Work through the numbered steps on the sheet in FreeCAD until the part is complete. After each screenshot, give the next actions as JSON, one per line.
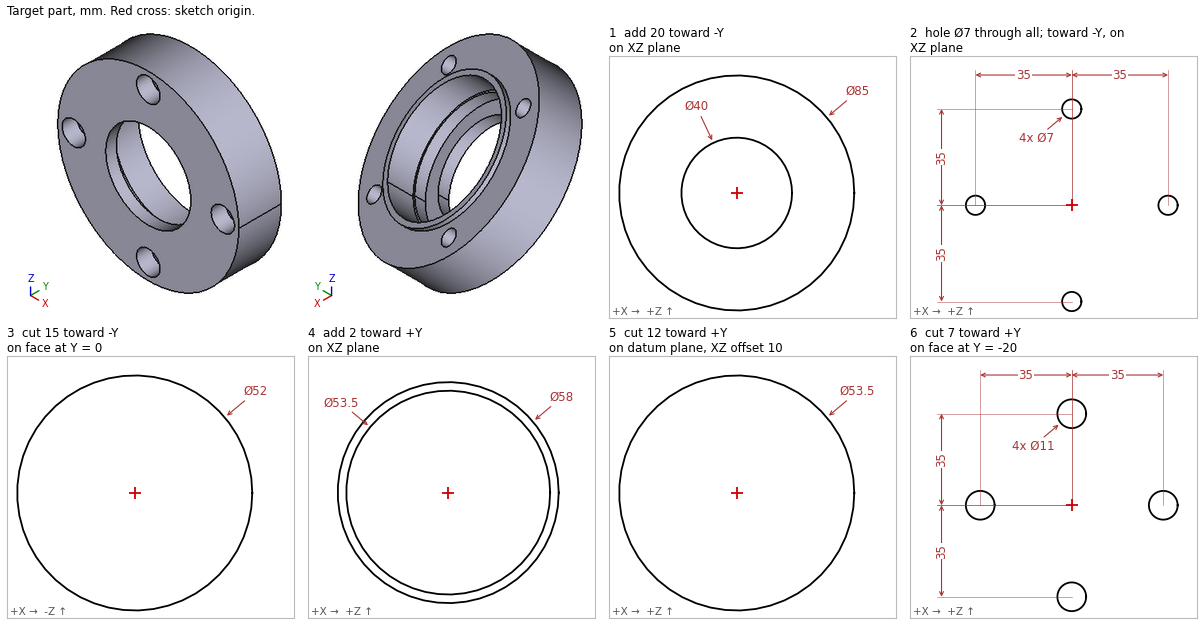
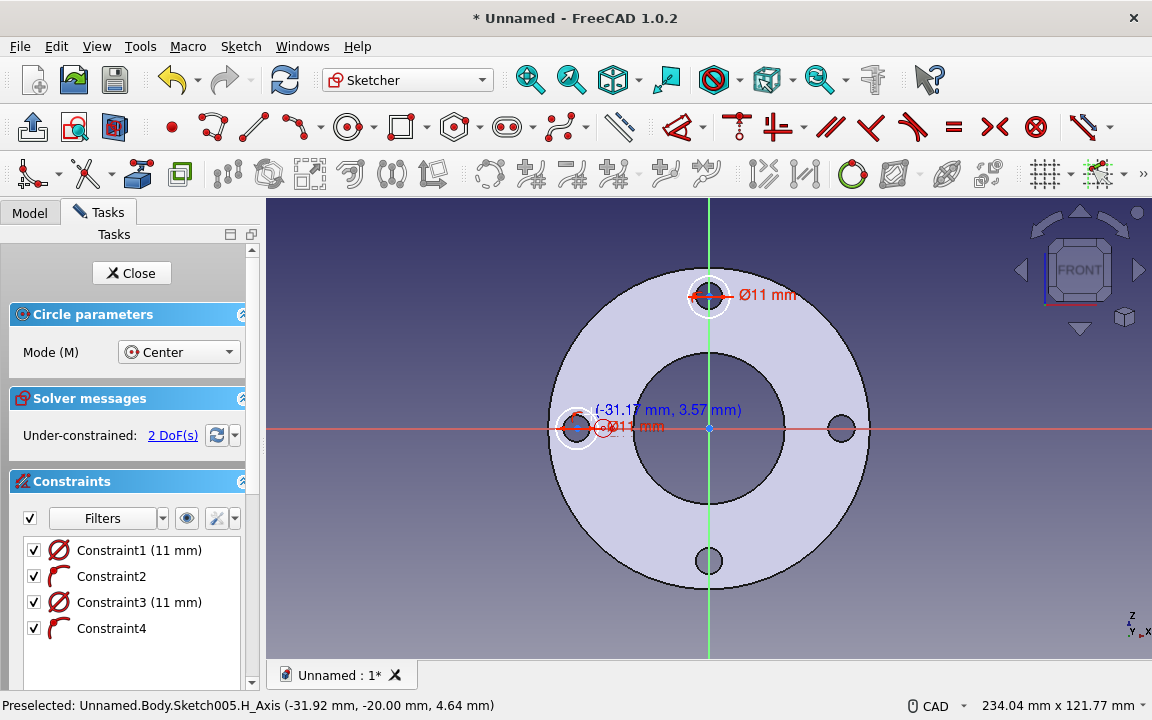
{"action": "left_click", "coordinate": [709, 561]}
{"action": "mouse_move", "coordinate": [724, 546]}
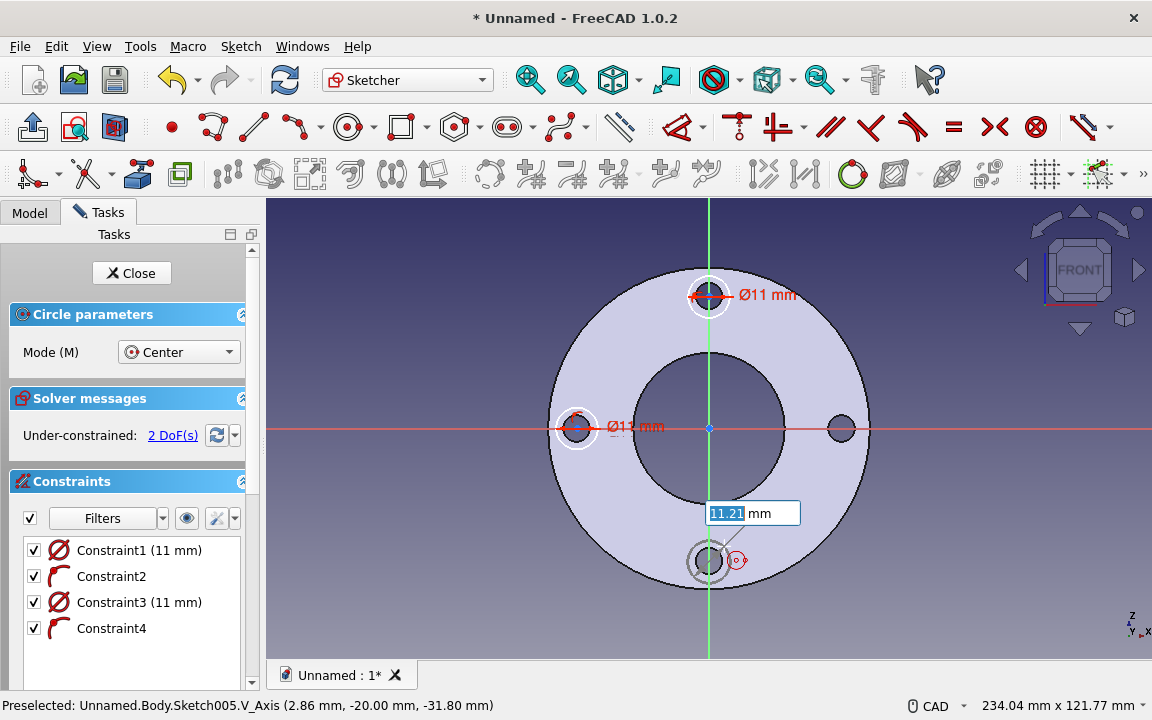
{"action": "type", "text": "11"}
{"action": "key", "text": "Return"}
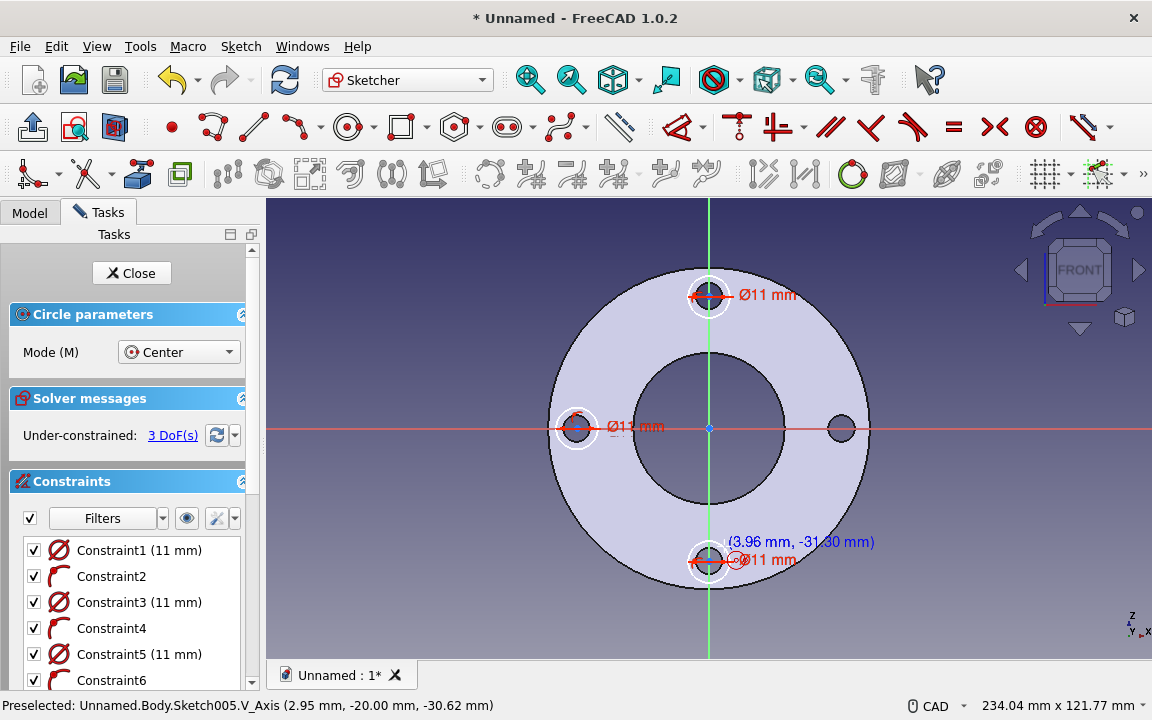
{"action": "left_click", "coordinate": [841, 428]}
{"action": "mouse_move", "coordinate": [856, 414]}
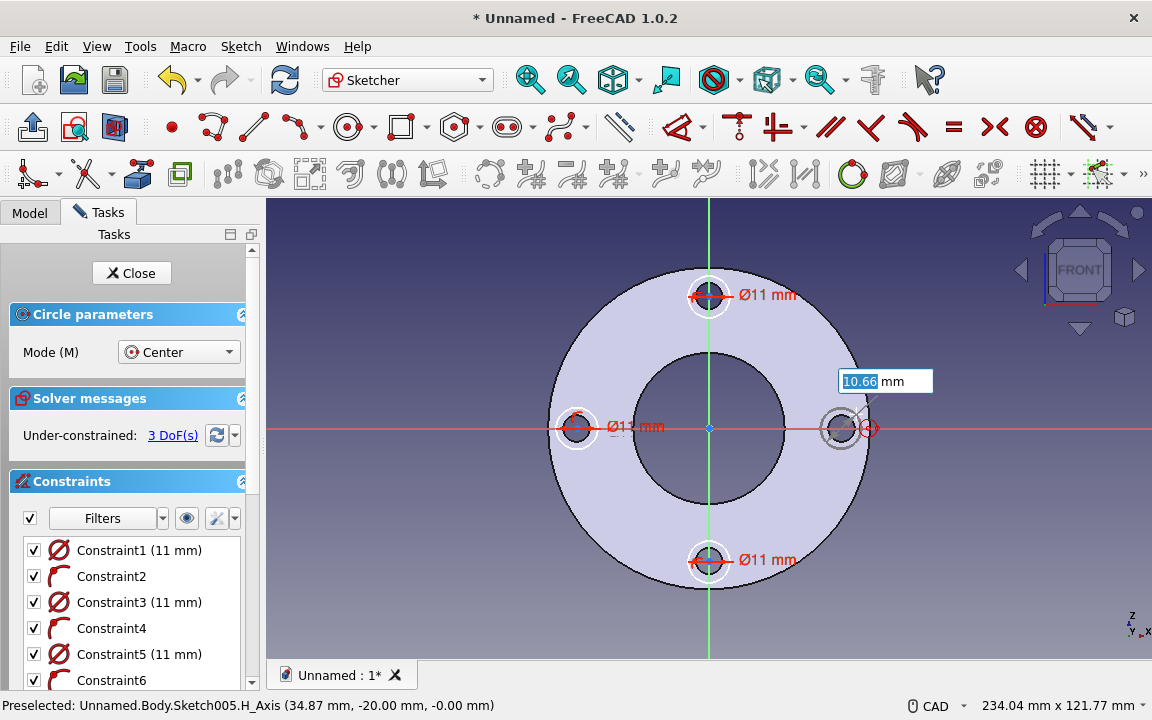
{"action": "type", "text": "11"}
{"action": "key", "text": "Return"}
{"action": "key", "text": "Escape"}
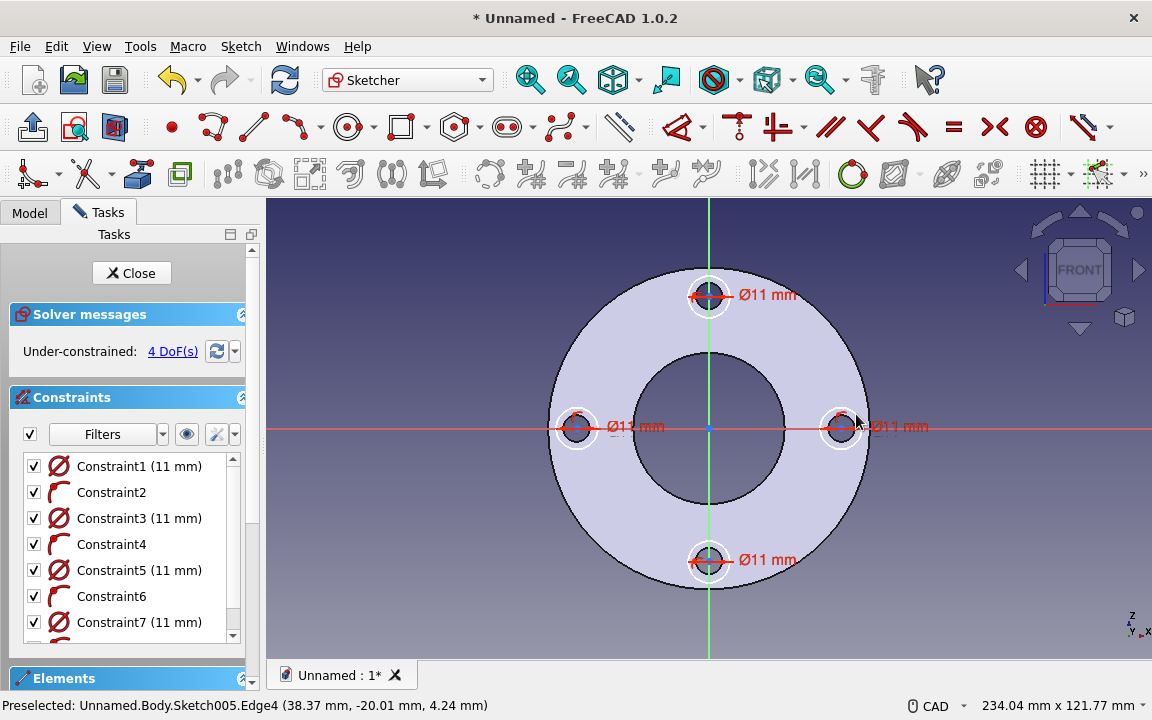
{"action": "left_click", "coordinate": [709, 297]}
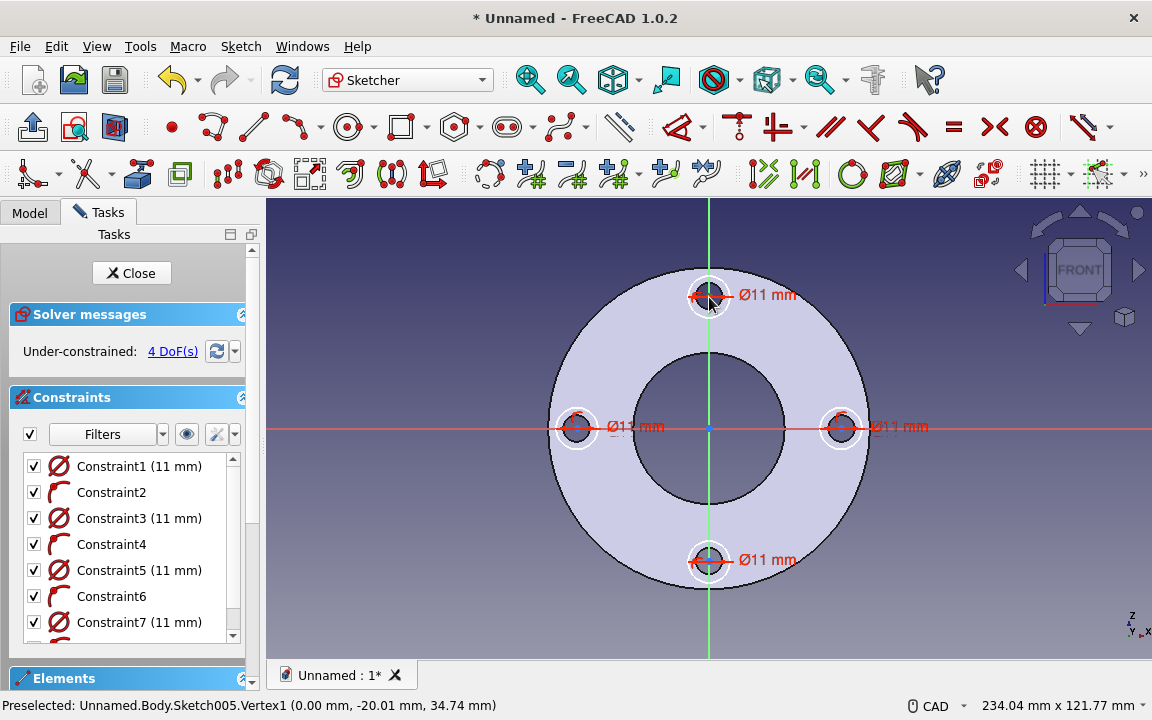
{"action": "key", "text": "i"}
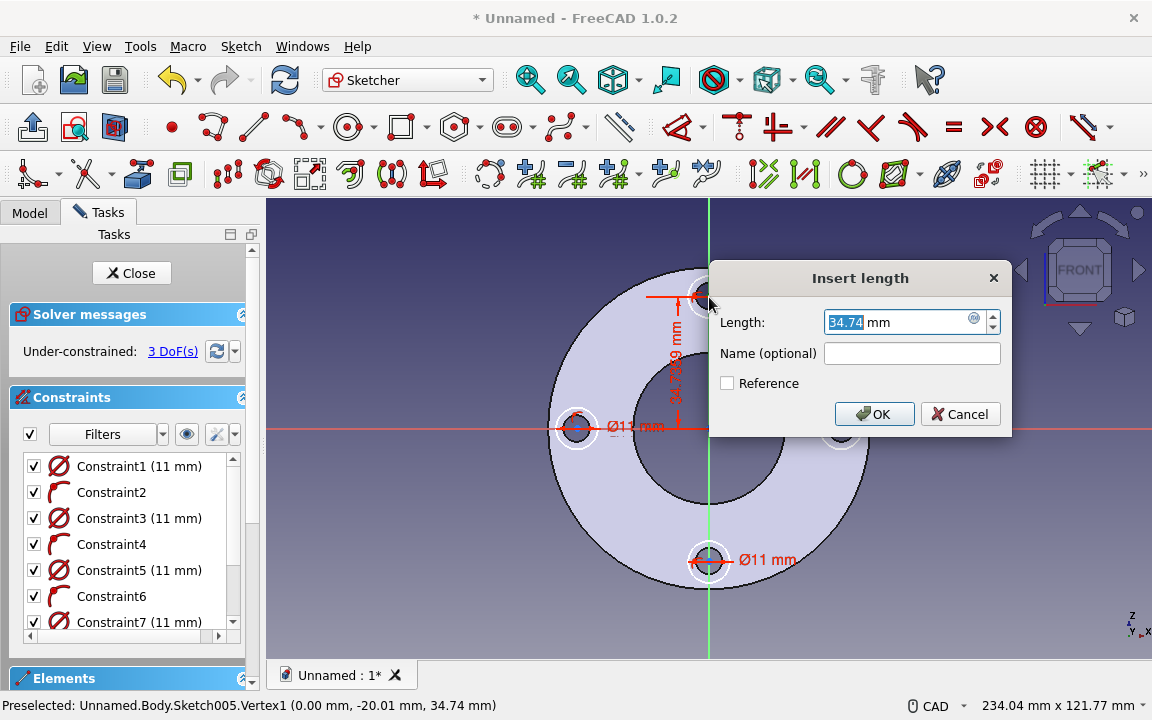
{"action": "type", "text": "35"}
{"action": "key", "text": "Return"}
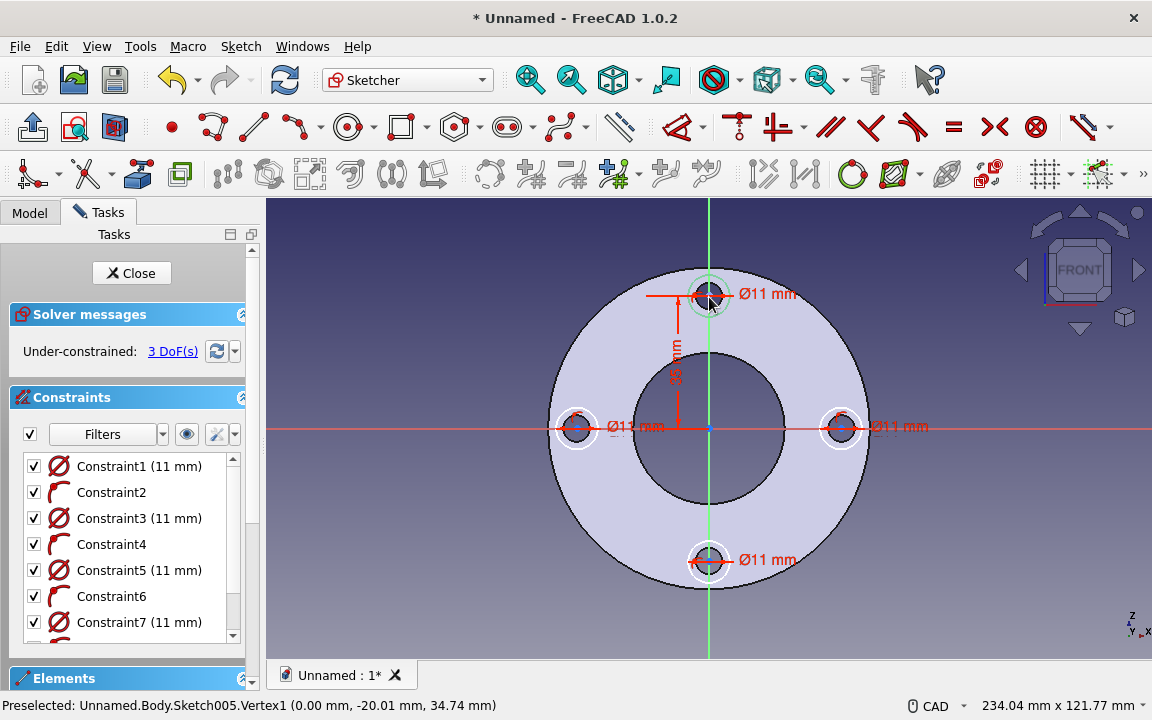
{"action": "left_click", "coordinate": [577, 428]}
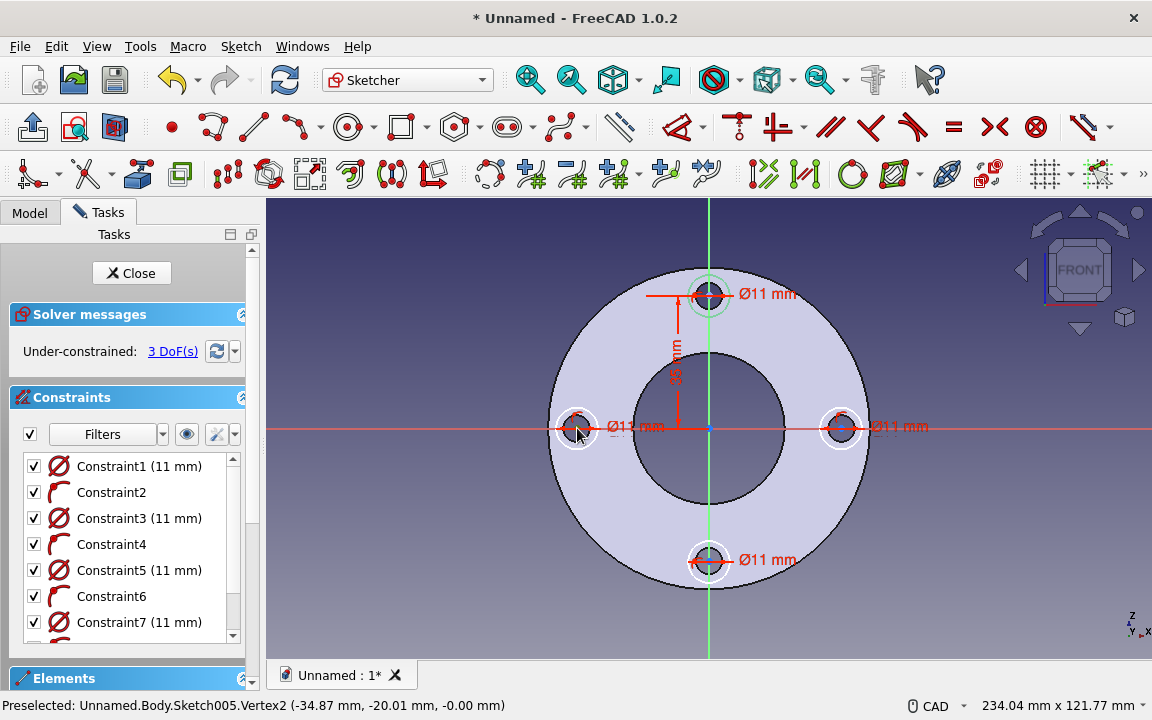
{"action": "key", "text": "l"}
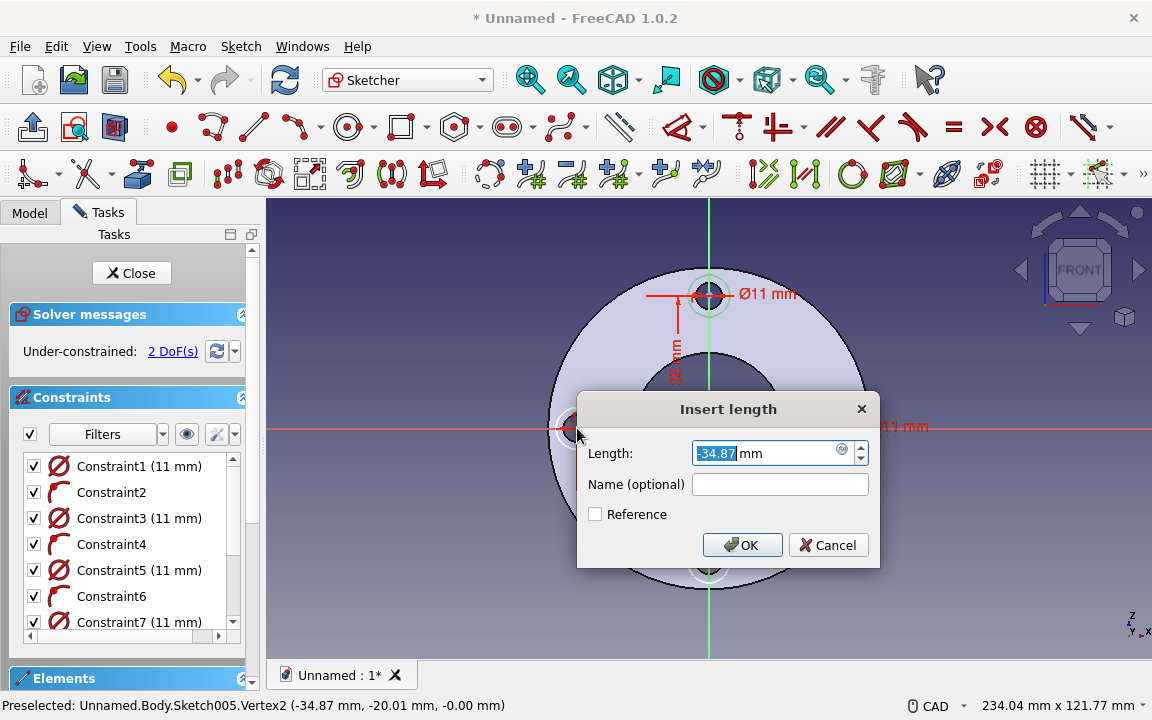
{"action": "type", "text": "-35"}
{"action": "key", "text": "Return"}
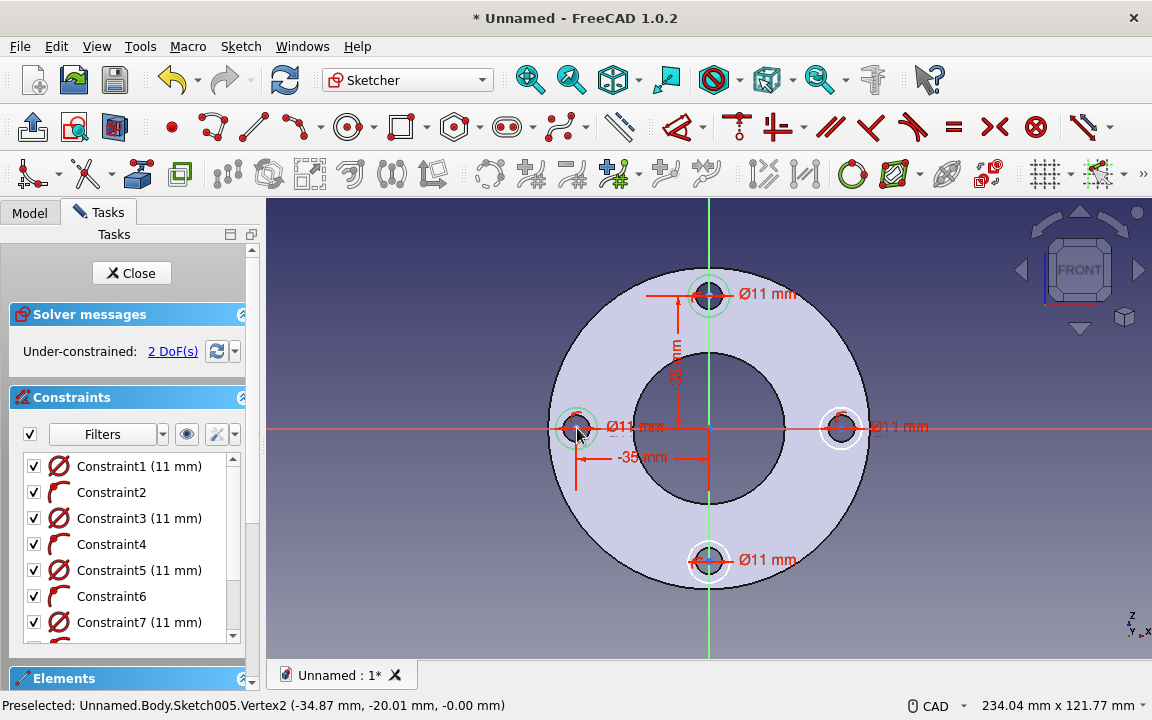
{"action": "left_click", "coordinate": [709, 562]}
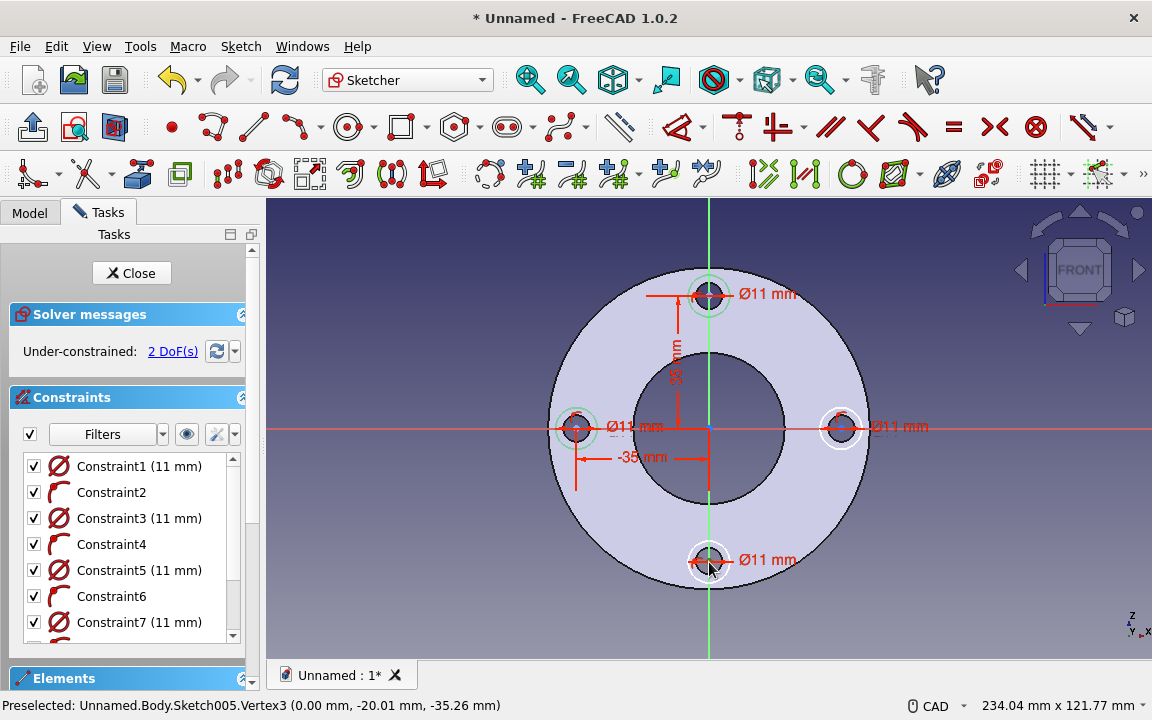
{"action": "key", "text": "i"}